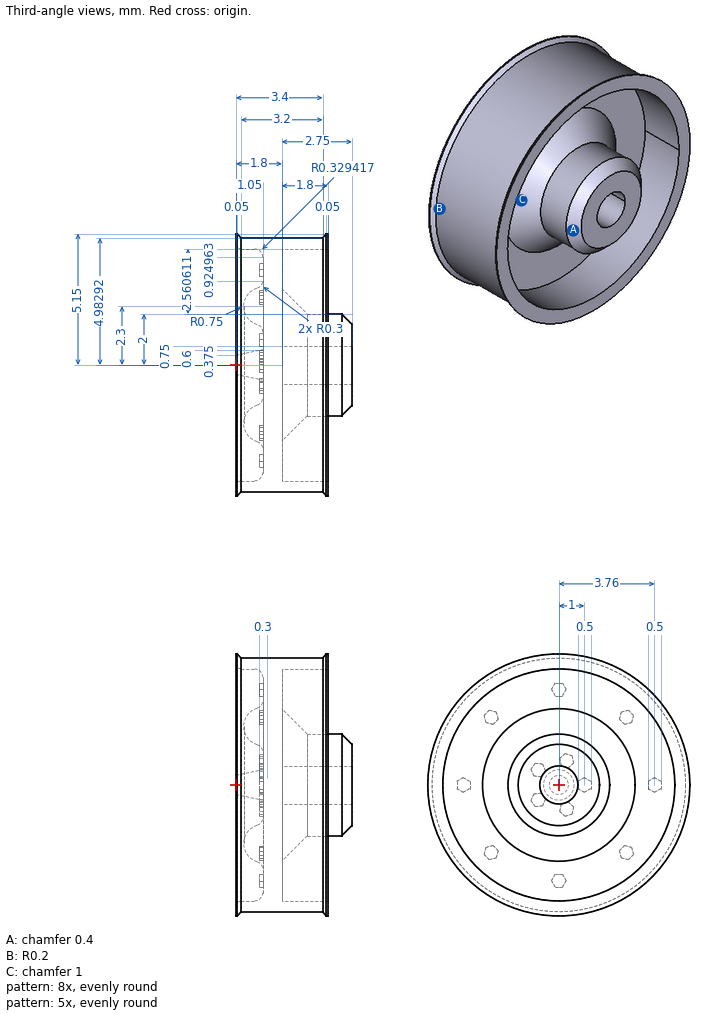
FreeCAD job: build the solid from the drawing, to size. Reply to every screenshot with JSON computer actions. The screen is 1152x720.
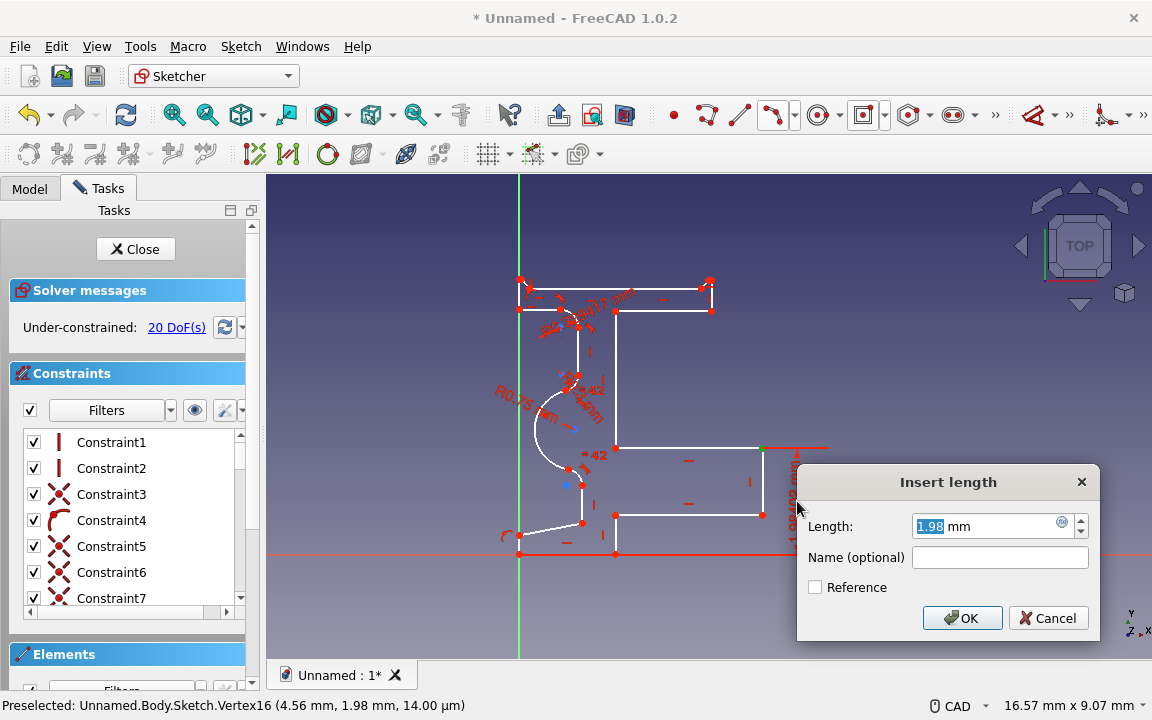
{"action": "type", "text": "2"}
{"action": "key", "text": "Return"}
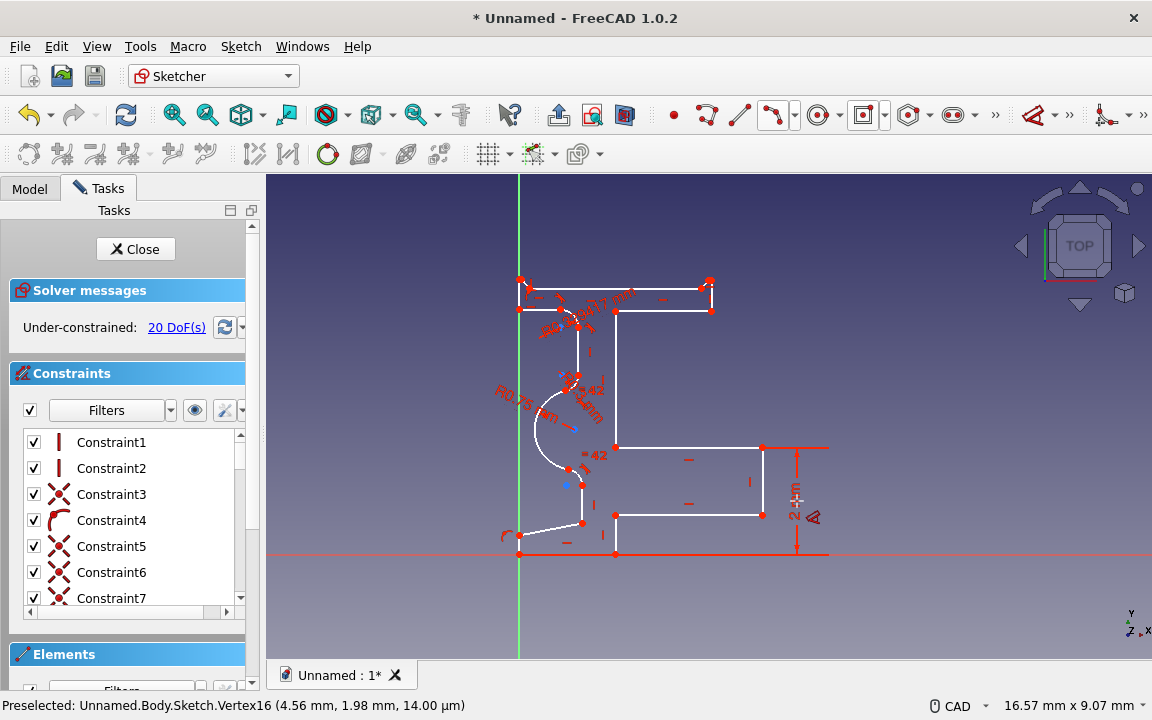
{"action": "left_click", "coordinate": [548, 555]}
{"action": "left_click", "coordinate": [568, 589]}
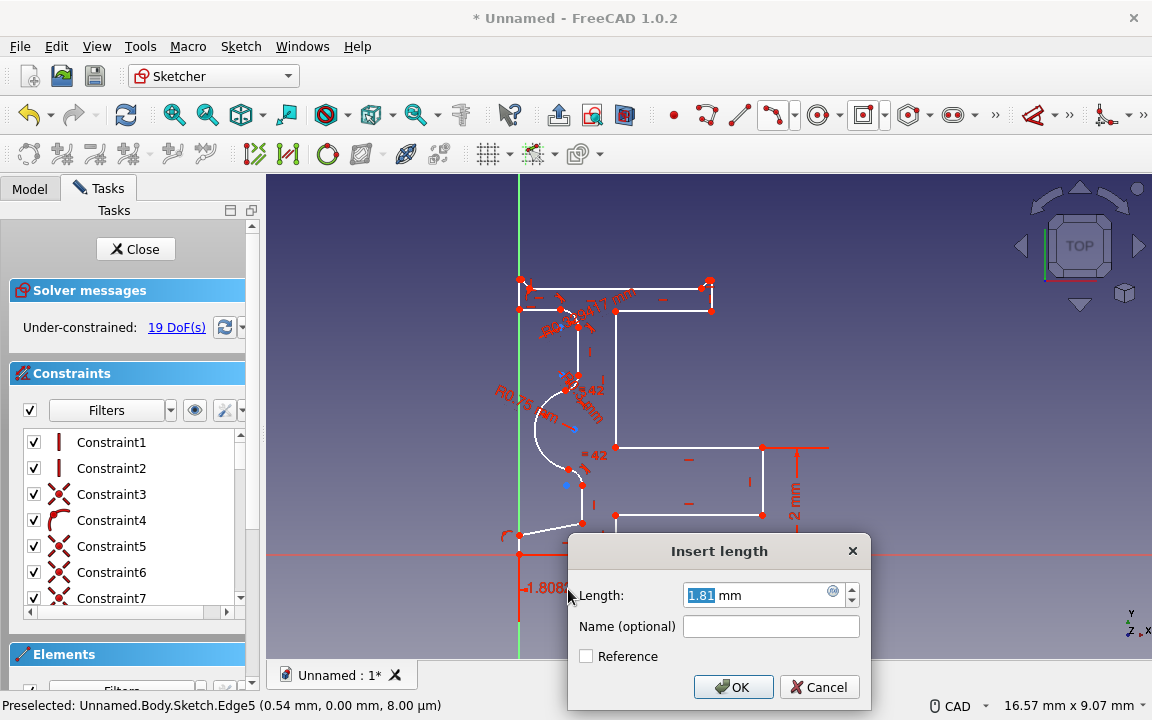
{"action": "type", "text": "1.8"}
{"action": "key", "text": "Return"}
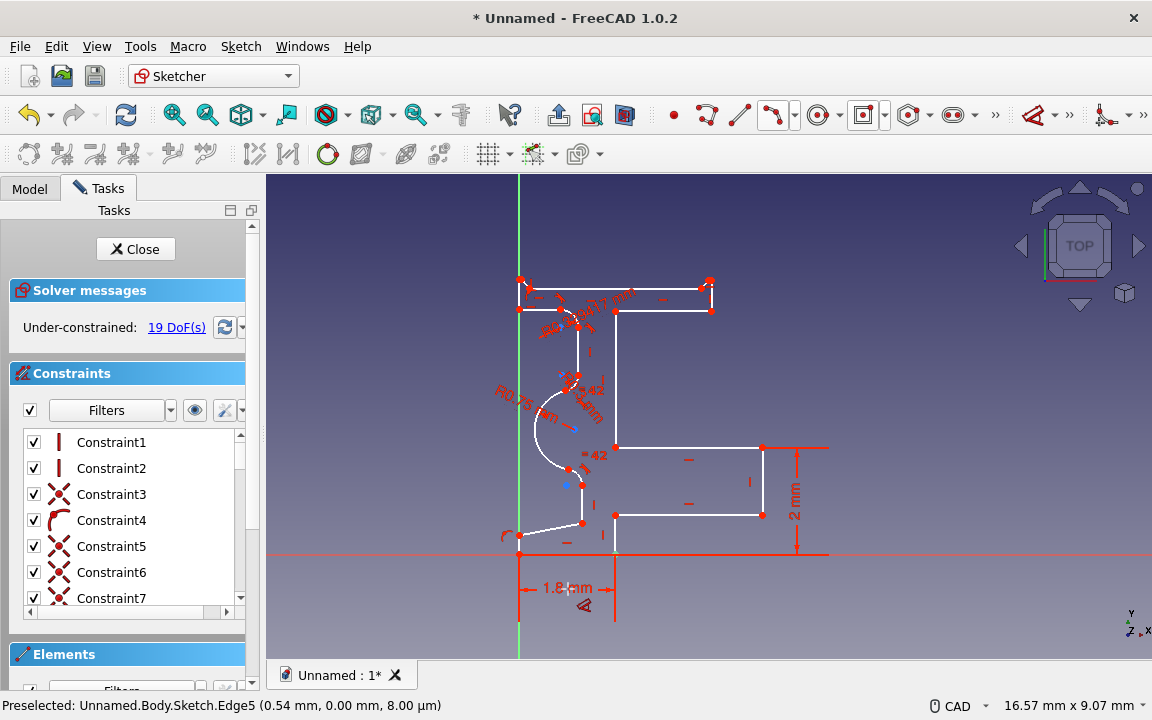
{"action": "left_click", "coordinate": [645, 311]}
{"action": "left_click", "coordinate": [664, 345]}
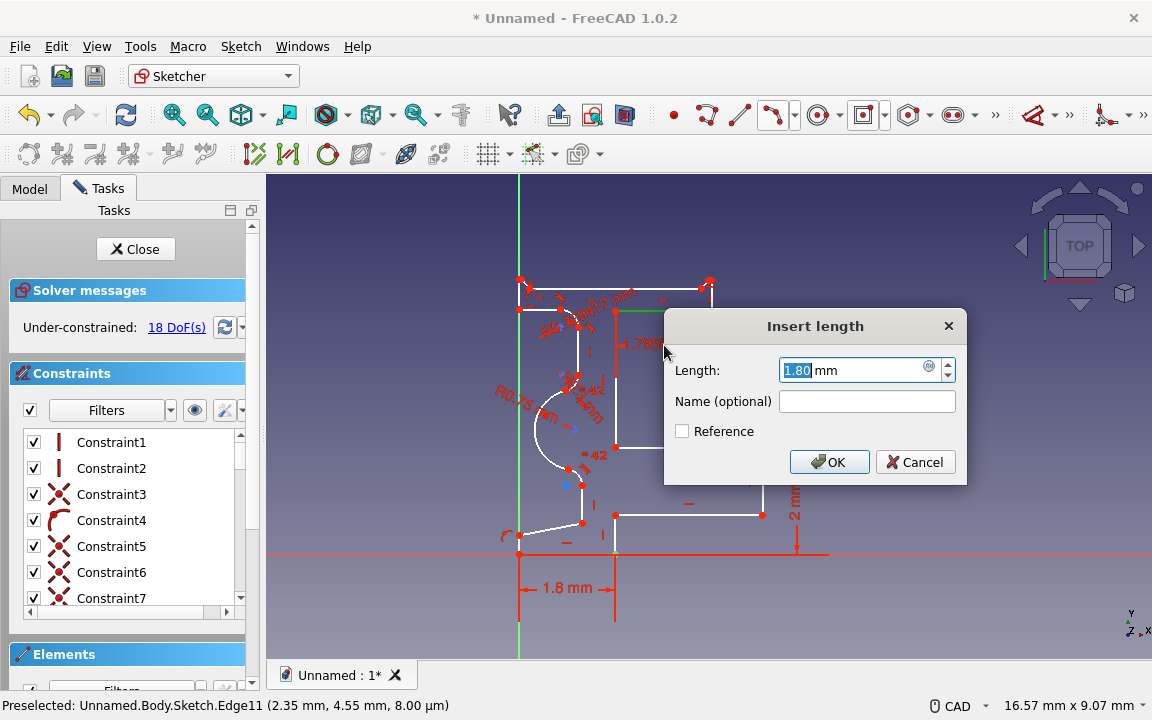
{"action": "type", "text": "1.8"}
{"action": "key", "text": "Return"}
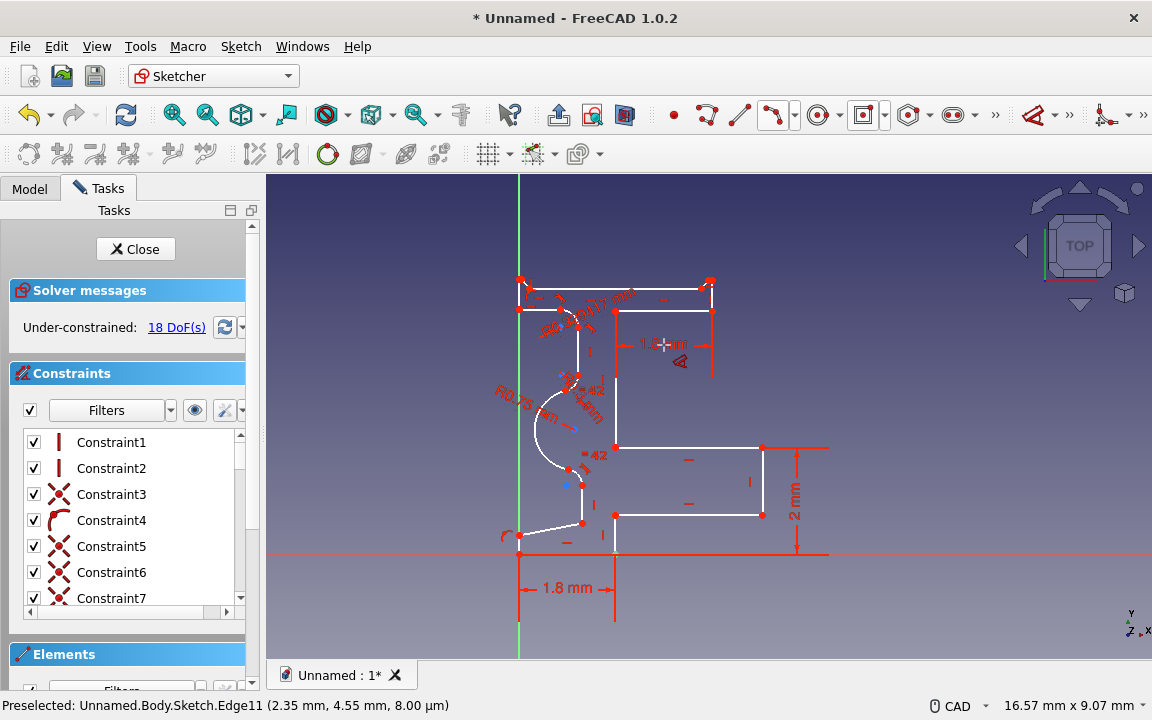
{"action": "left_click", "coordinate": [650, 289]}
{"action": "left_click", "coordinate": [615, 255]}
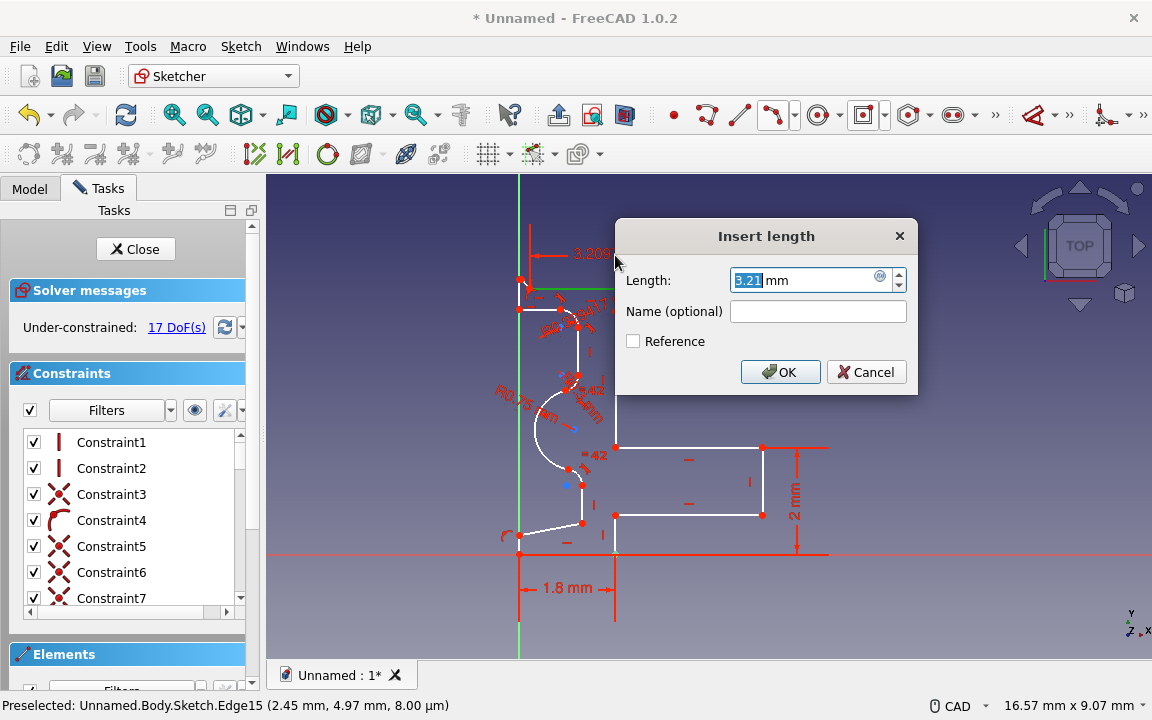
{"action": "type", "text": "3.2"}
{"action": "key", "text": "Return"}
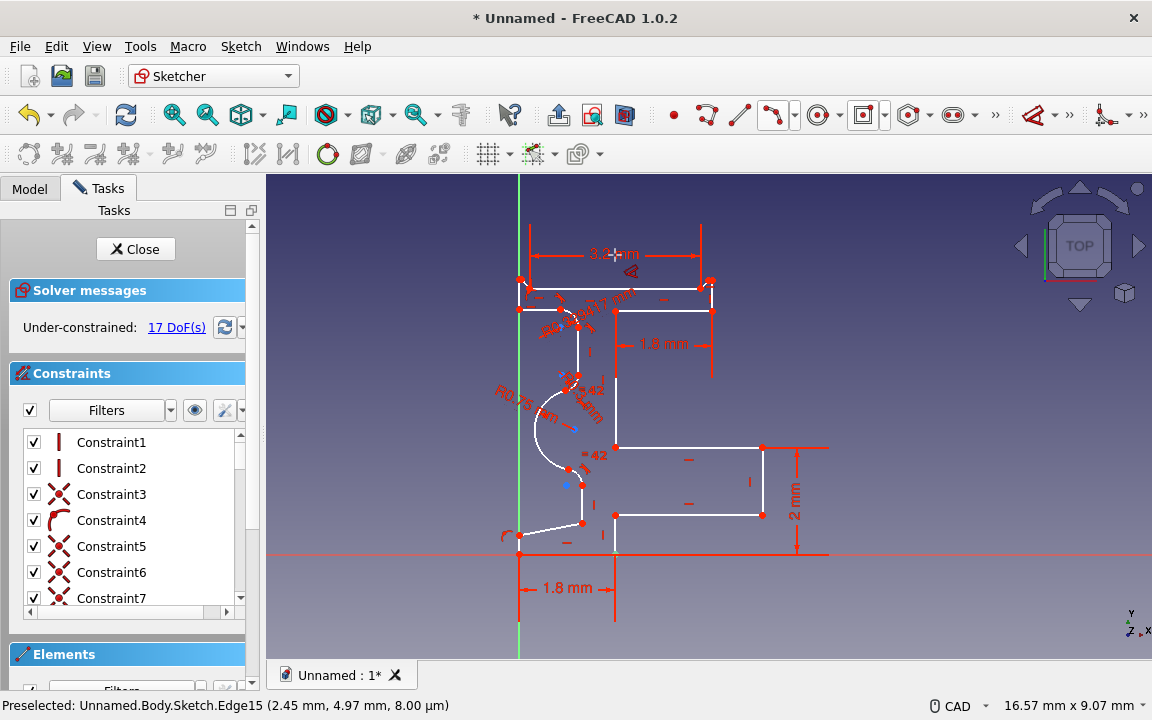
{"action": "left_click", "coordinate": [615, 543]}
{"action": "left_click", "coordinate": [649, 535]}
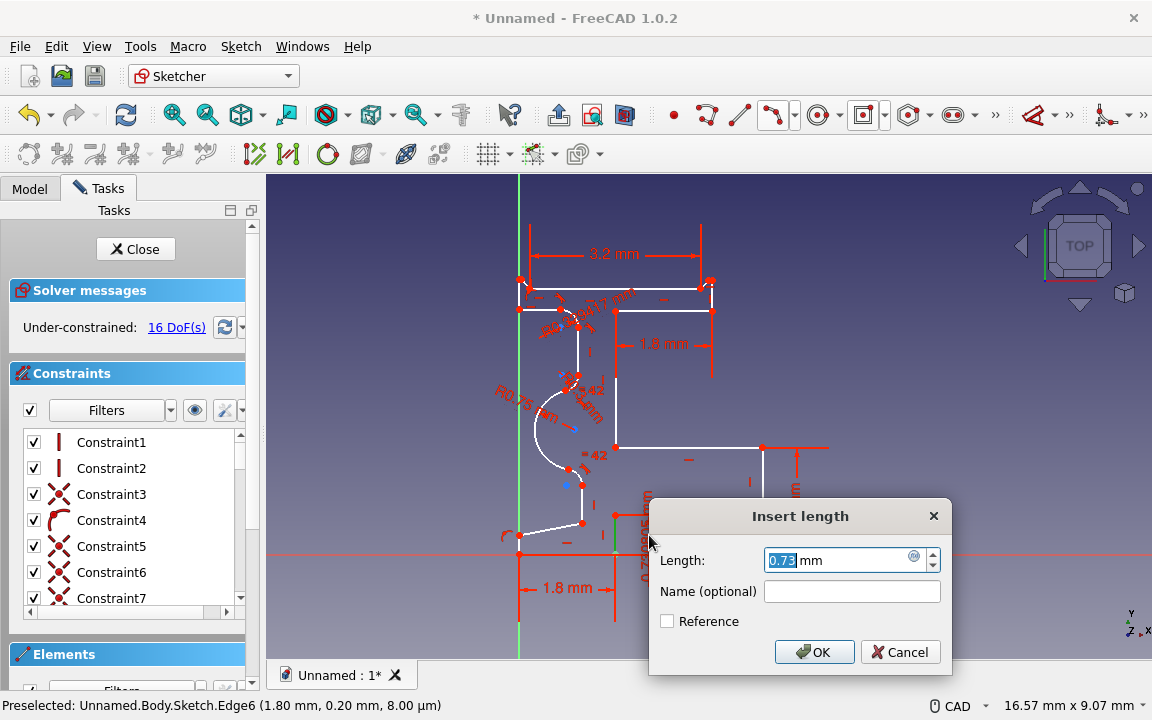
{"action": "type", "text": "0.75"}
{"action": "key", "text": "Return"}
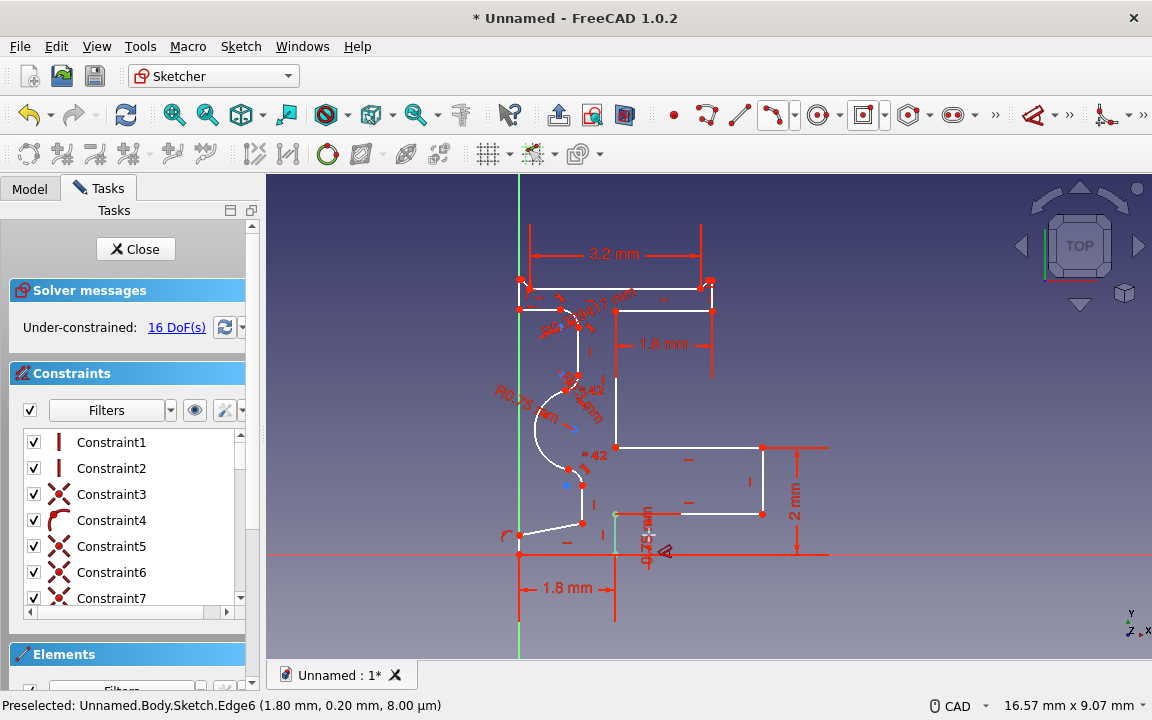
{"action": "left_click", "coordinate": [660, 514]}
{"action": "left_click", "coordinate": [689, 480]}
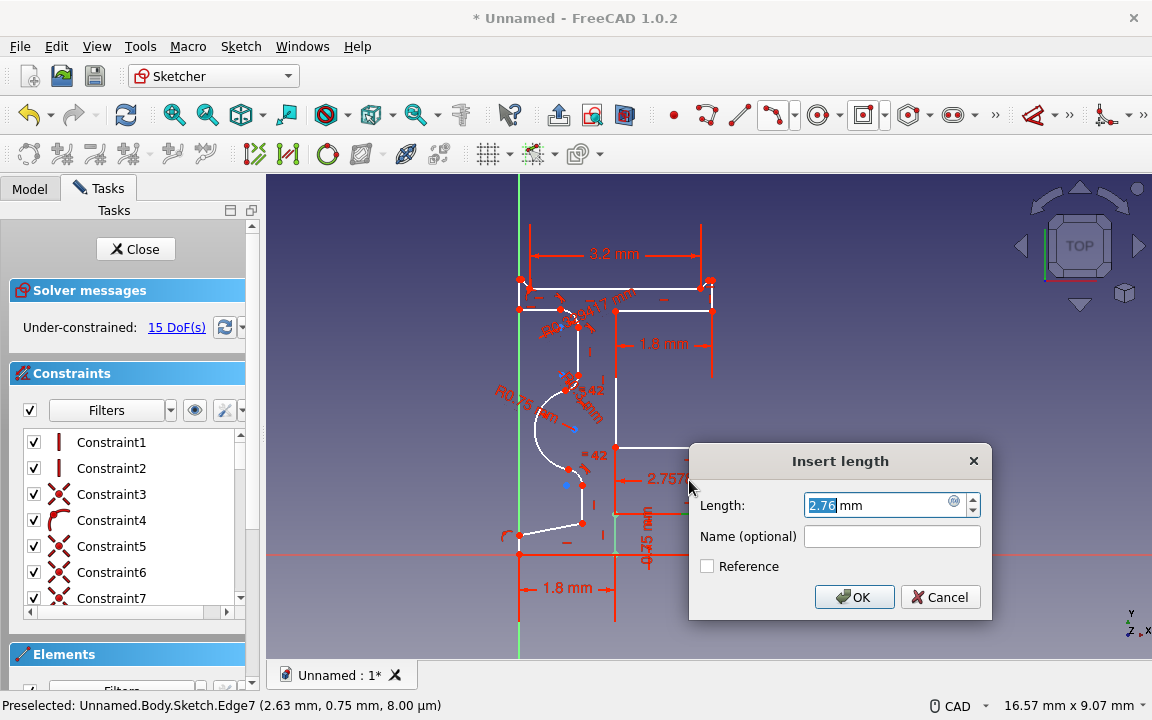
{"action": "type", "text": "2.75"}
{"action": "key", "text": "Return"}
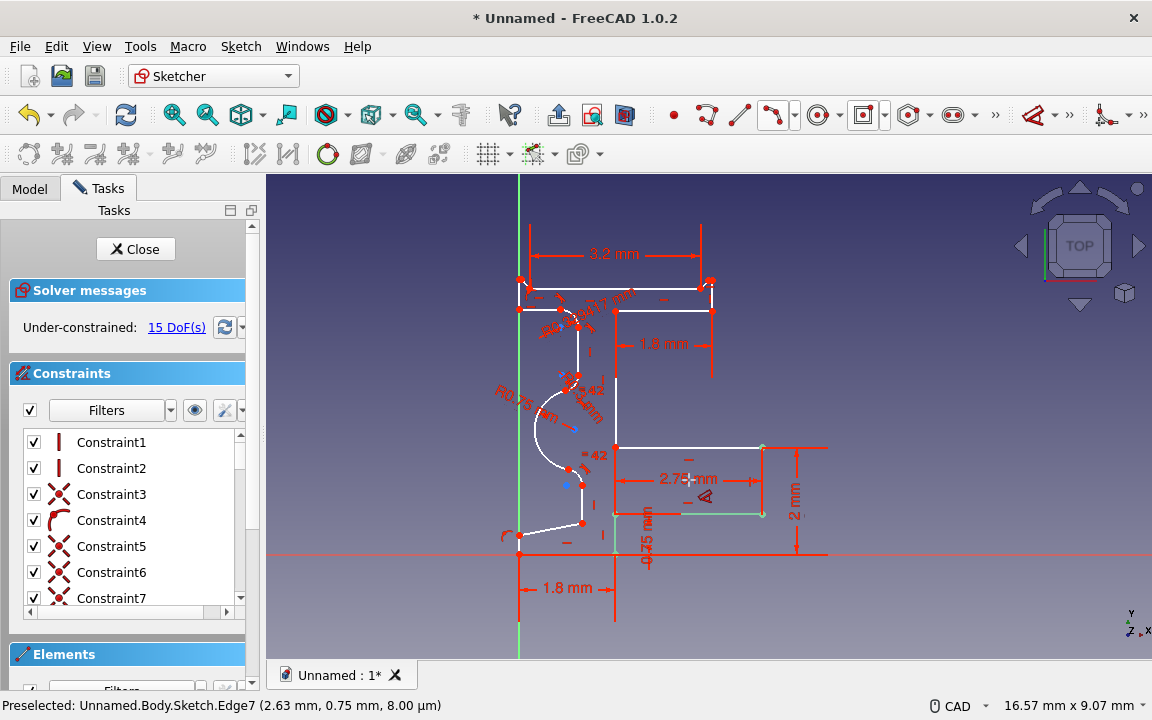
{"action": "left_click", "coordinate": [719, 448]}
{"action": "left_click", "coordinate": [689, 414]}